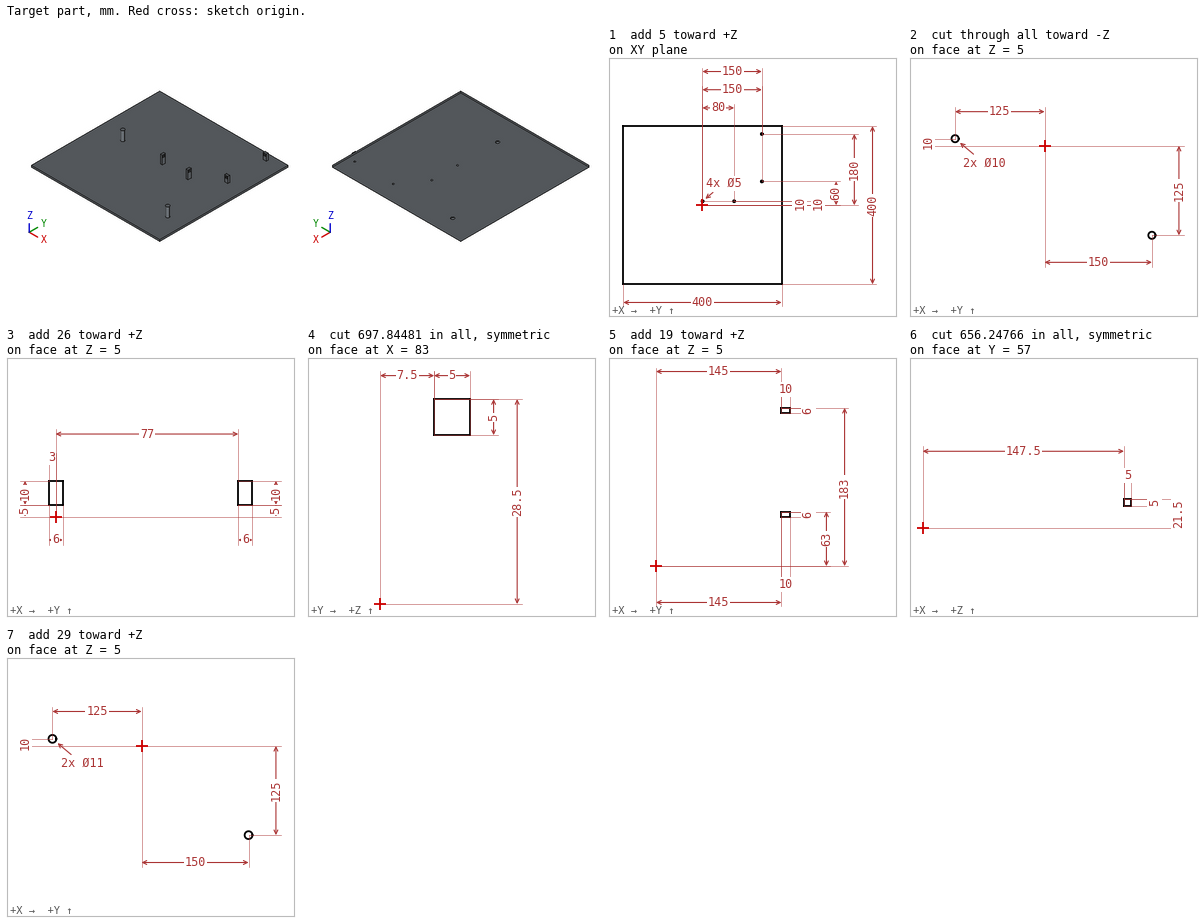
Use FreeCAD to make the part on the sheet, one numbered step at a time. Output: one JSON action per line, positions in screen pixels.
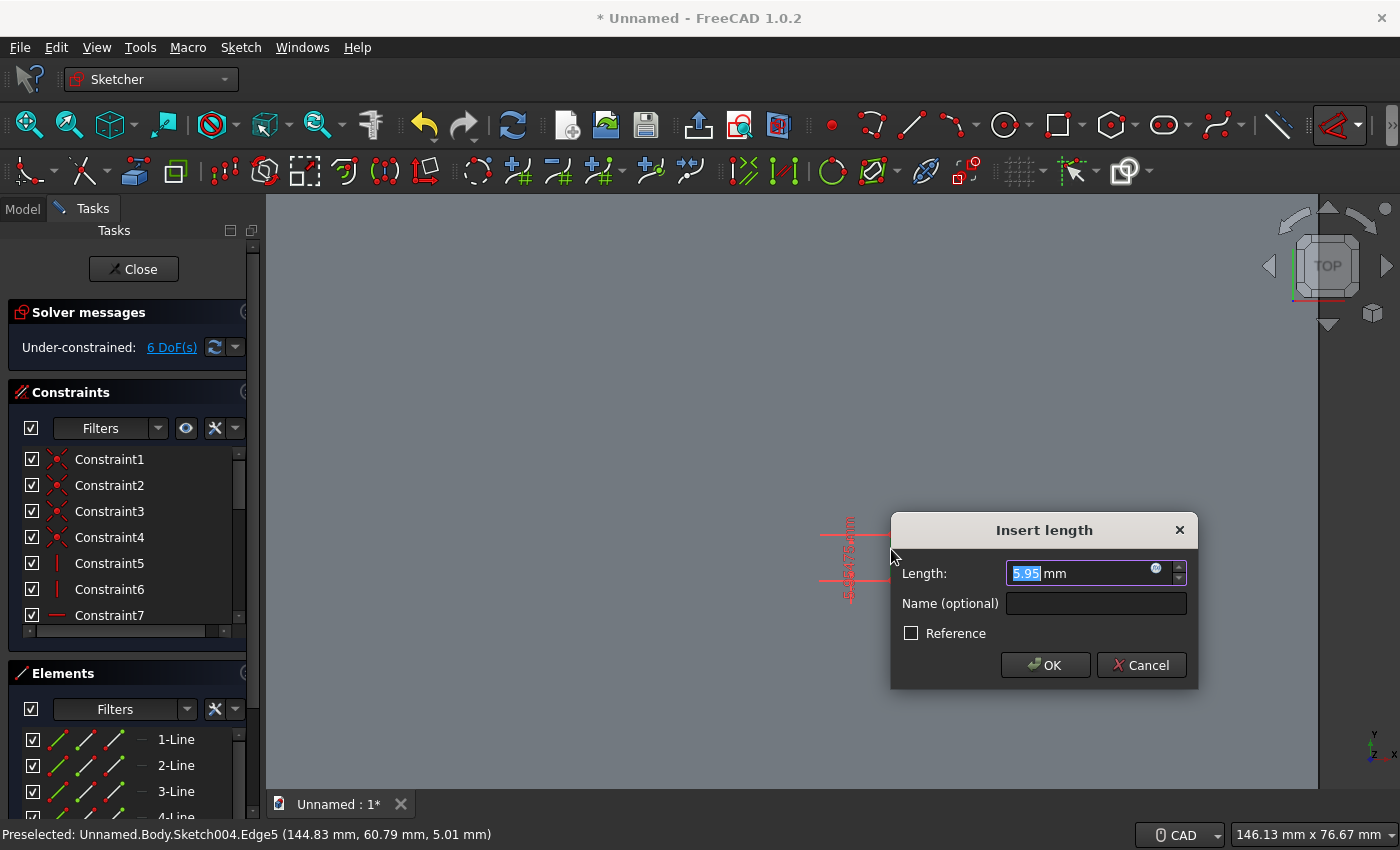
{"action": "type", "text": "6"}
{"action": "key", "text": "Return"}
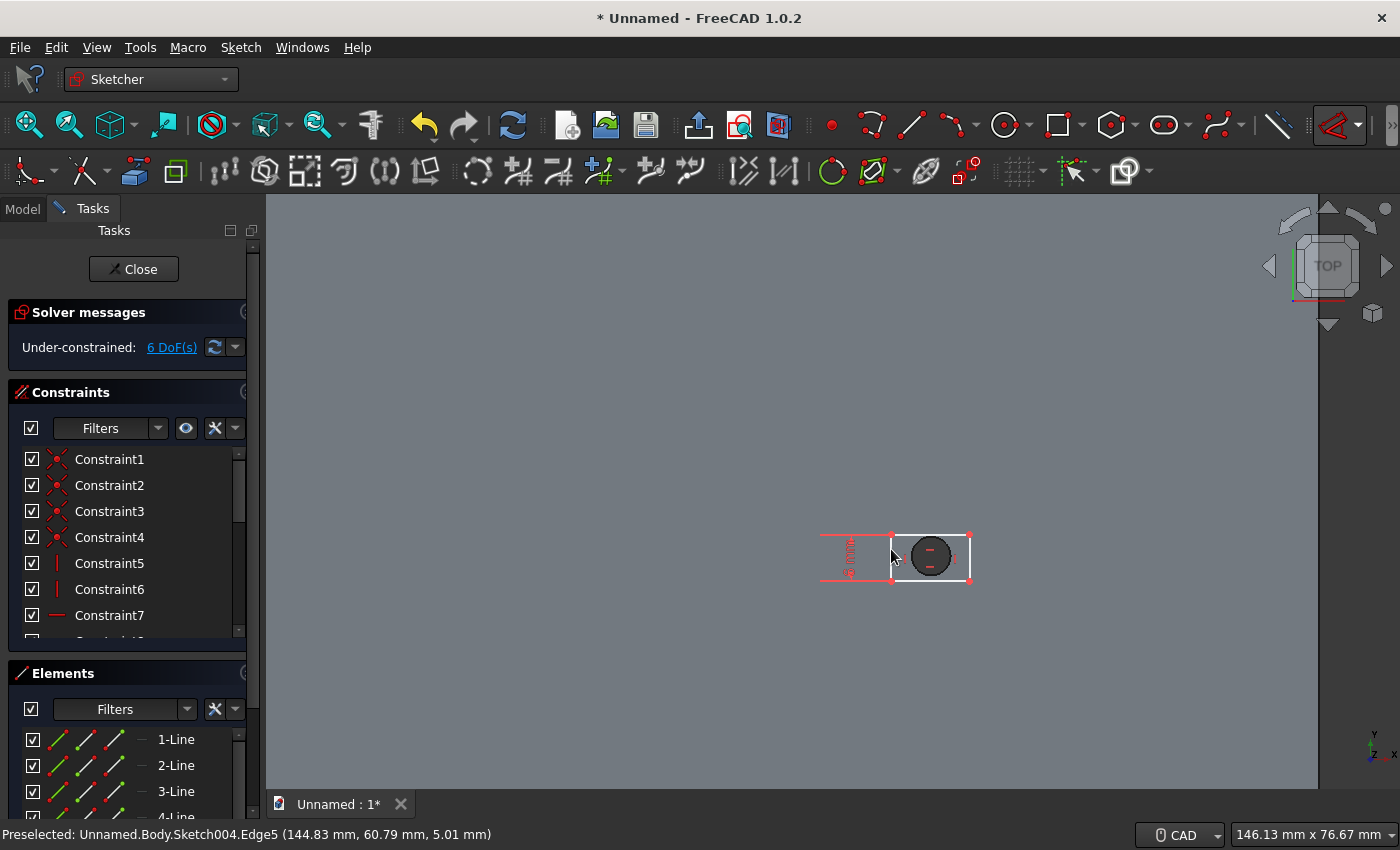
{"action": "scroll", "coordinate": [894, 550], "scroll_direction": "down", "scroll_amount": 7}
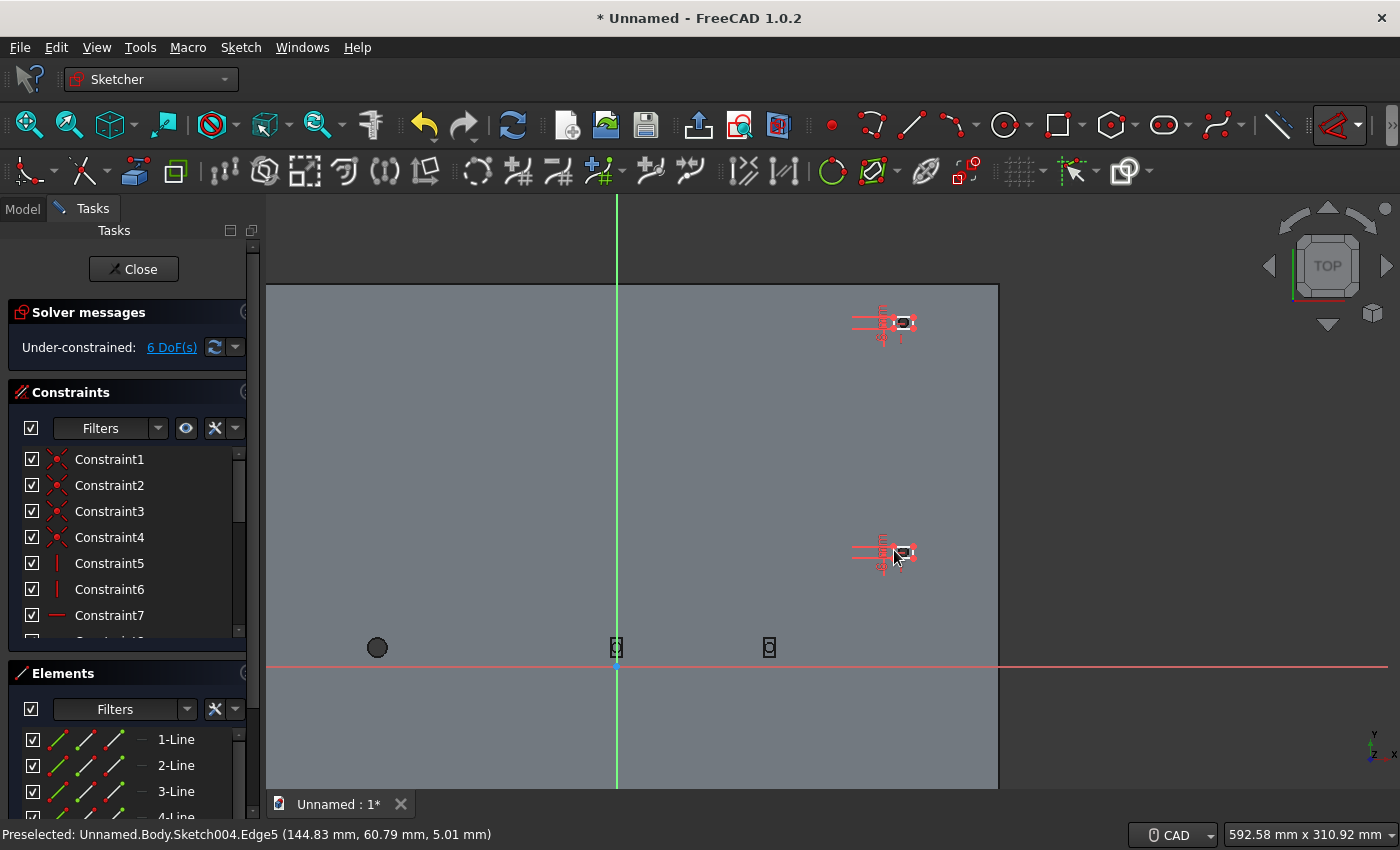
{"action": "scroll", "coordinate": [900, 329], "scroll_direction": "up", "scroll_amount": 5}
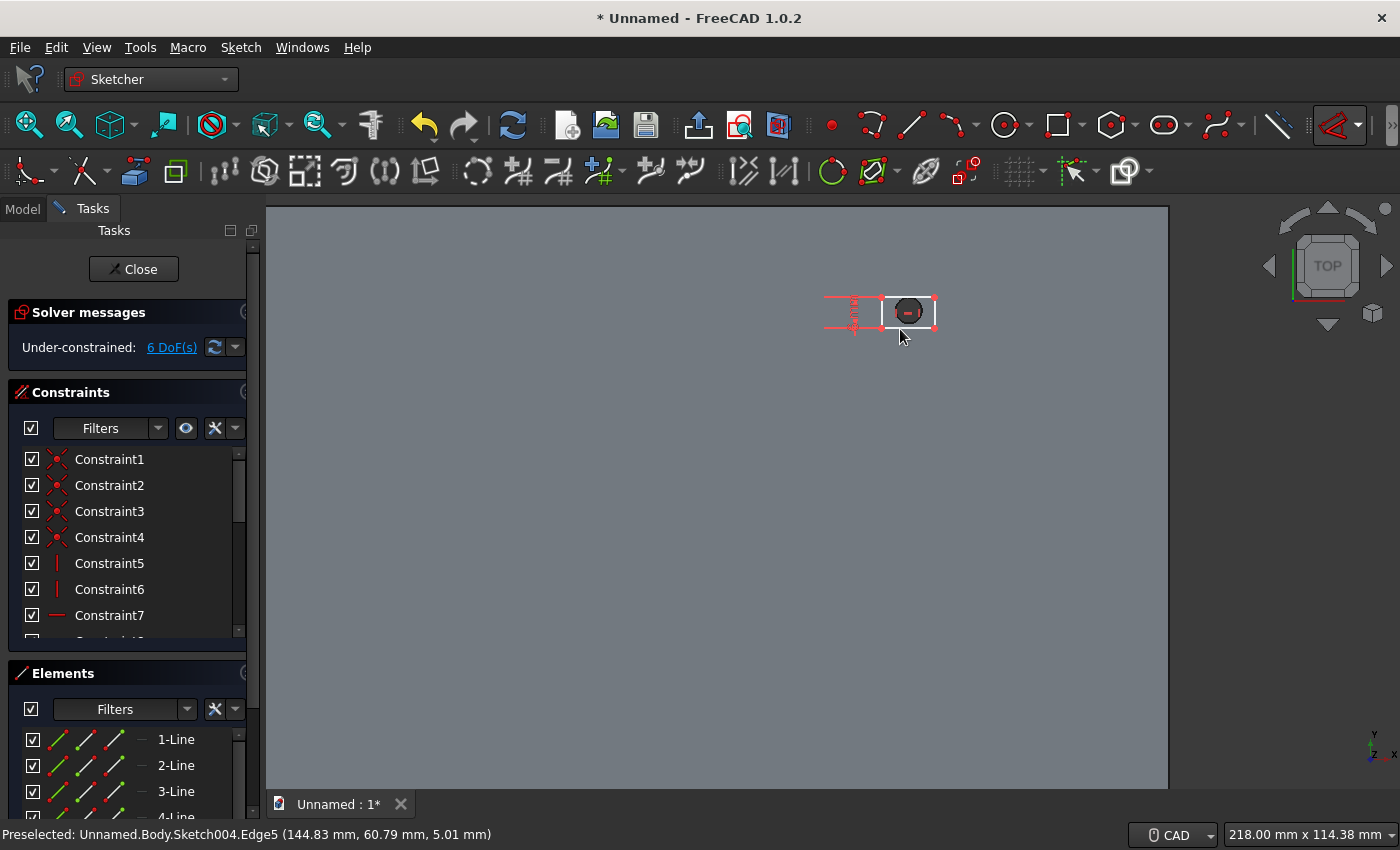
{"action": "left_click", "coordinate": [898, 328]}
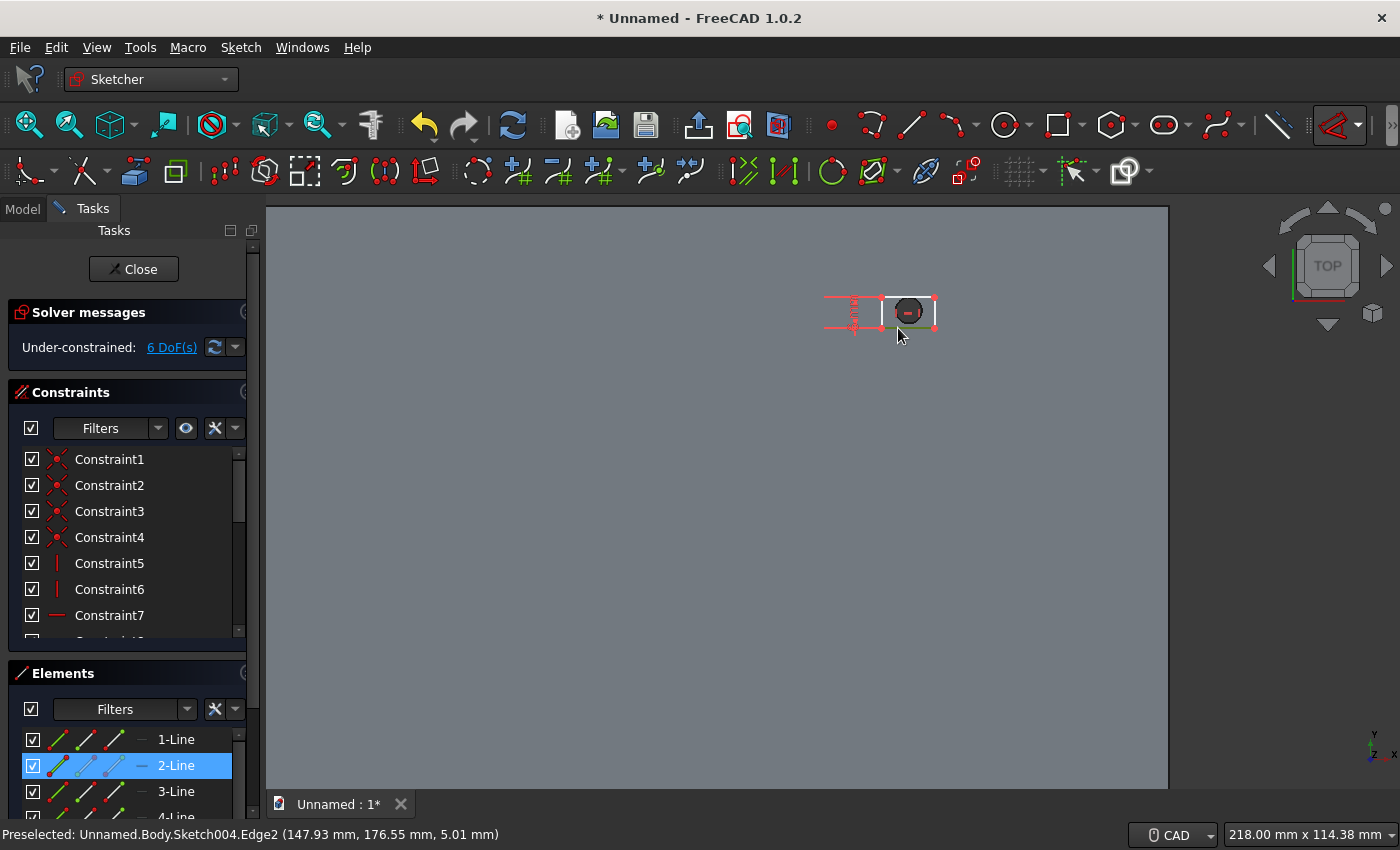
{"action": "key", "text": "l"}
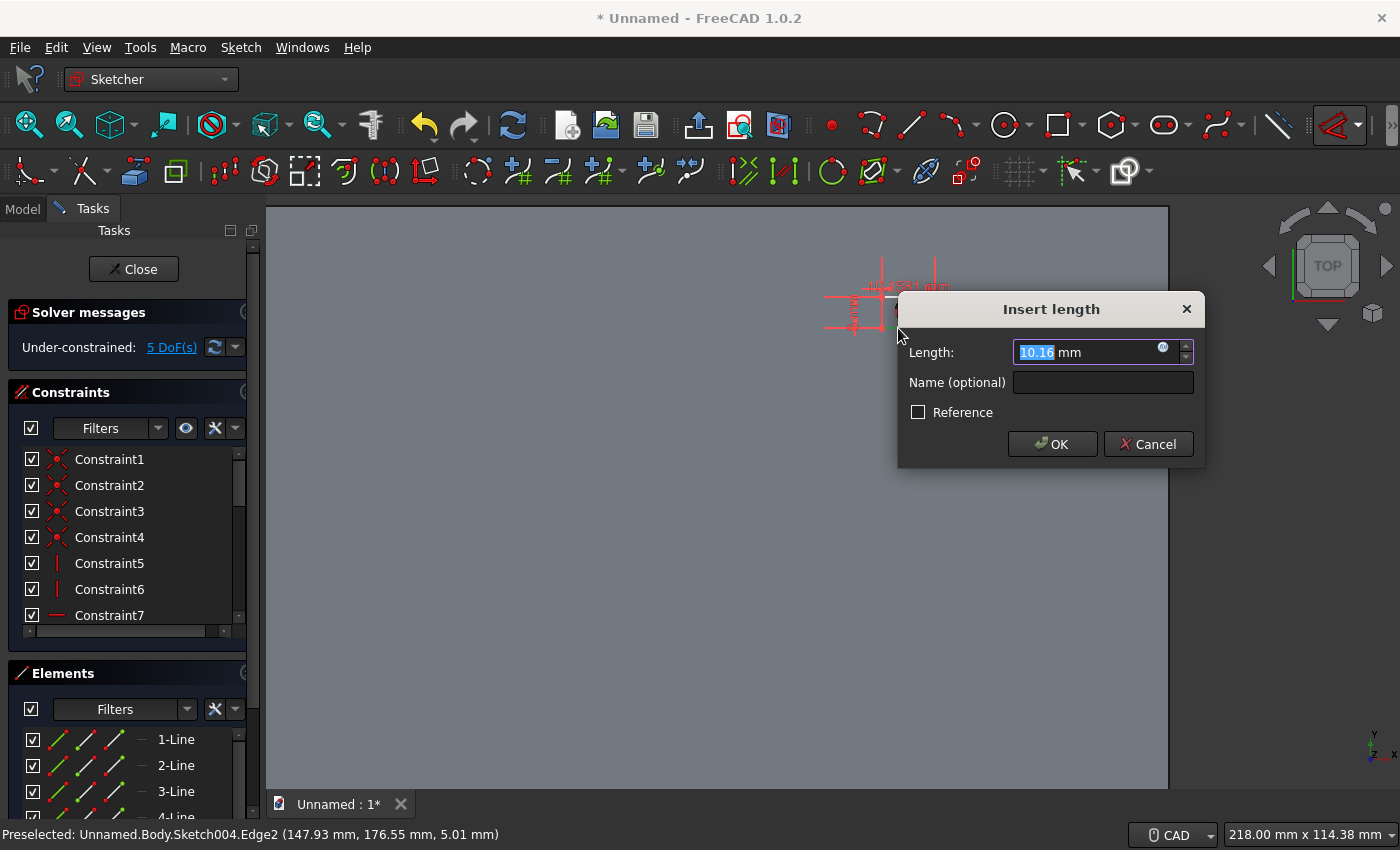
{"action": "type", "text": "10"}
{"action": "key", "text": "Return"}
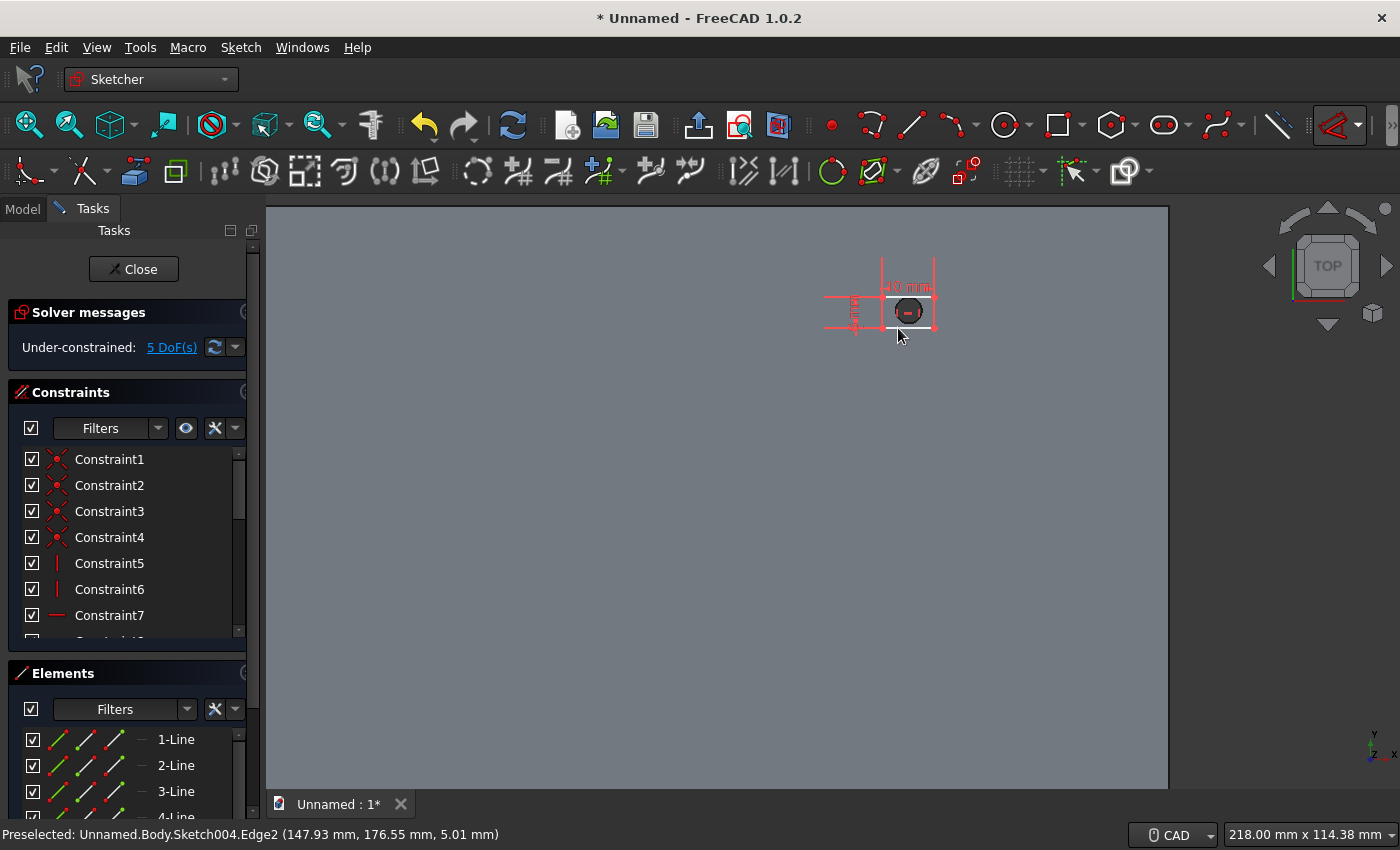
{"action": "scroll", "coordinate": [900, 329], "scroll_direction": "down", "scroll_amount": 5}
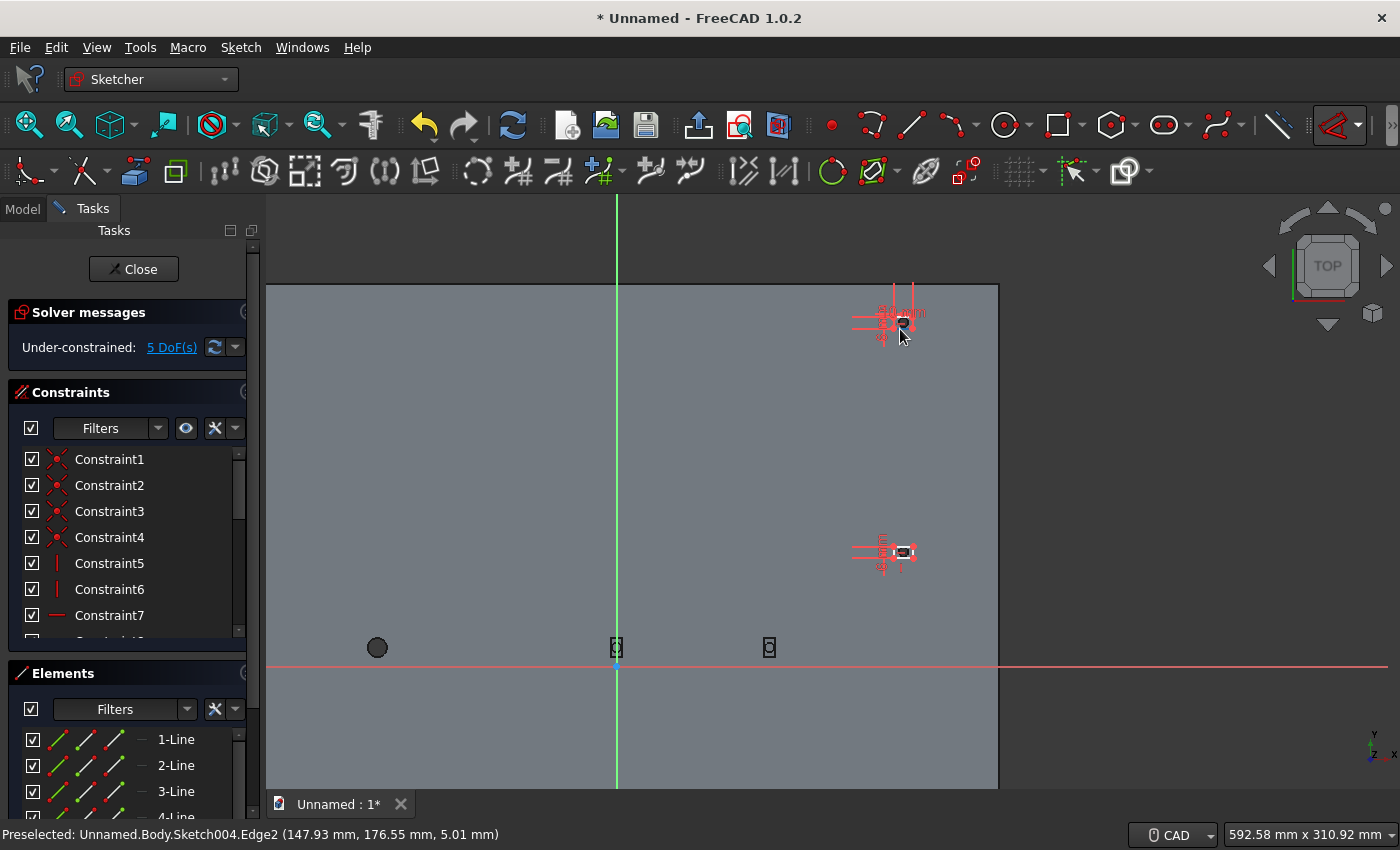
{"action": "scroll", "coordinate": [900, 558], "scroll_direction": "up", "scroll_amount": 5}